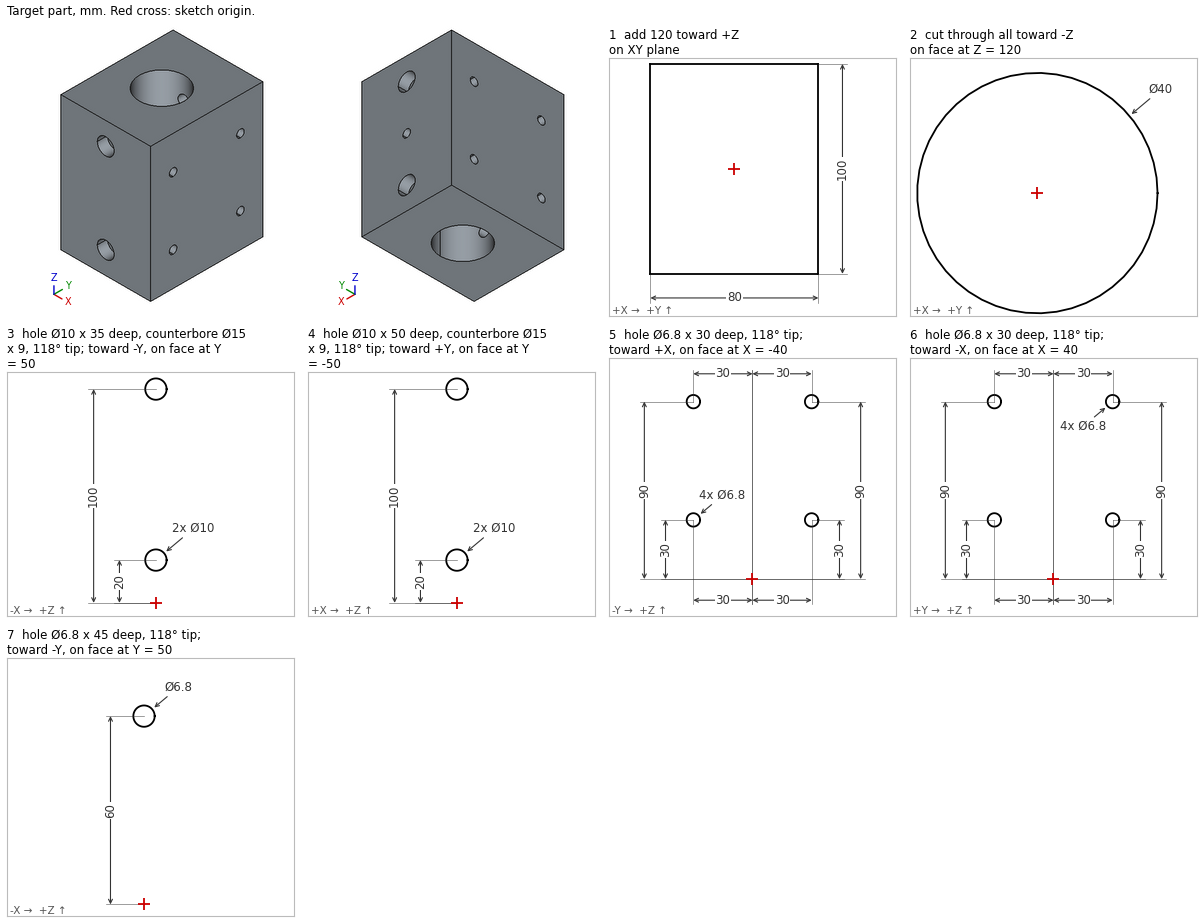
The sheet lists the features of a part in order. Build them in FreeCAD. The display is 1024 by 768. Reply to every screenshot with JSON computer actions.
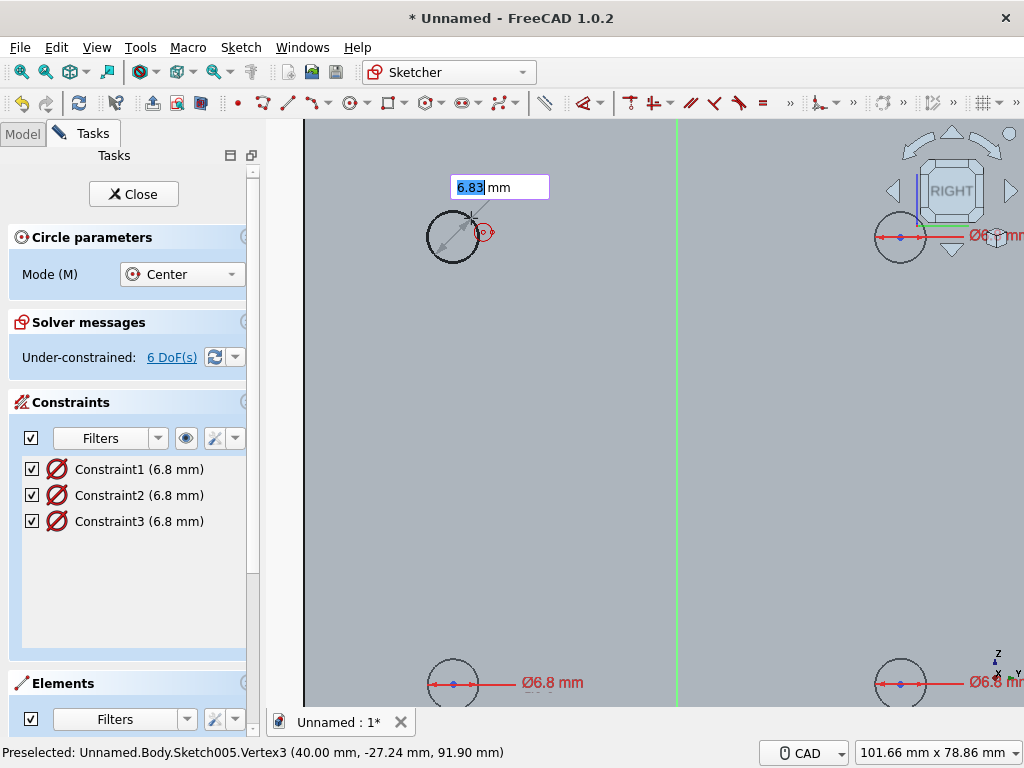
{"action": "type", "text": "6.8"}
{"action": "key", "text": "Return"}
{"action": "key", "text": "Escape"}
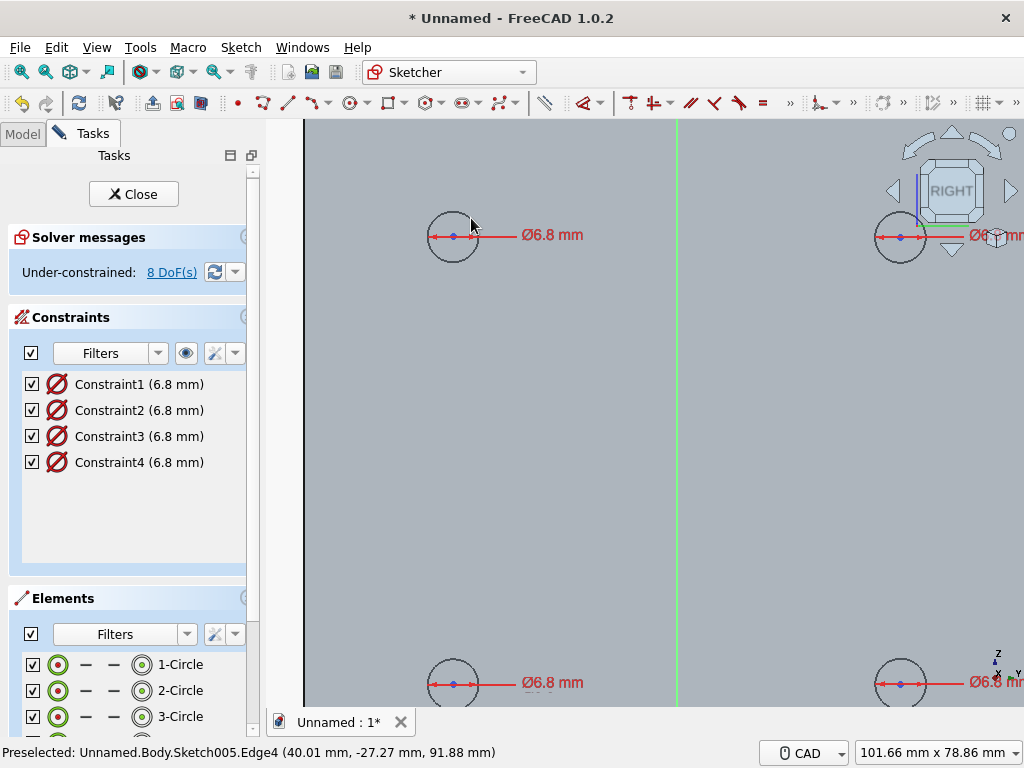
{"action": "left_click", "coordinate": [584, 104]}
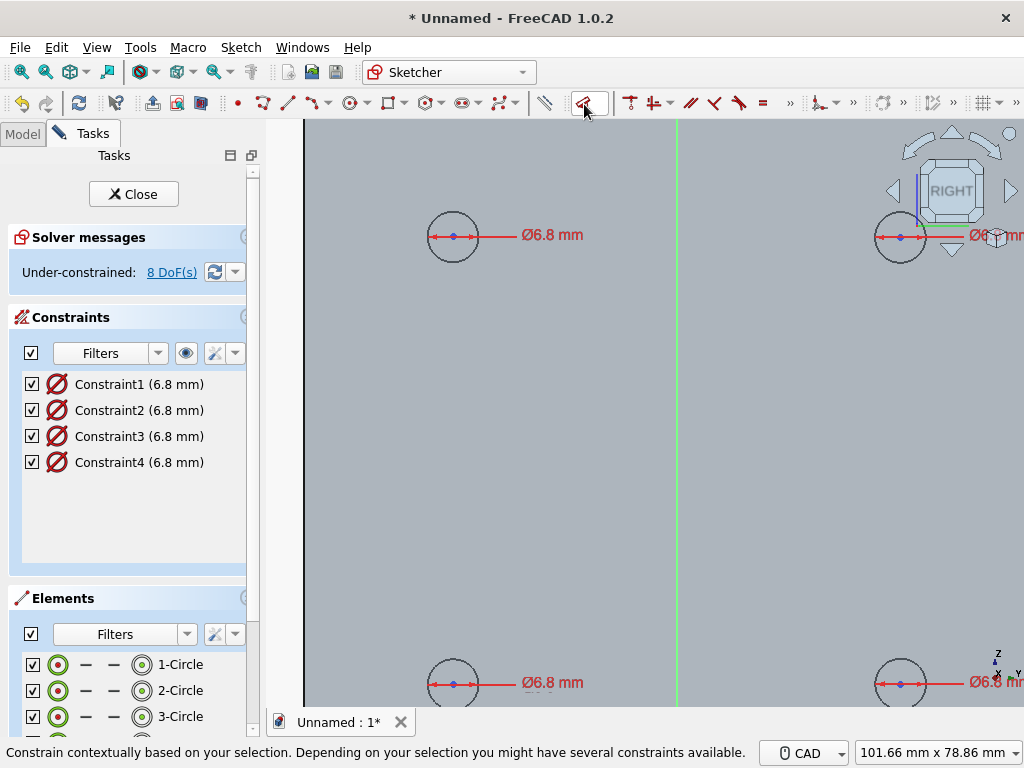
{"action": "scroll", "coordinate": [454, 235], "scroll_direction": "down", "scroll_amount": 3}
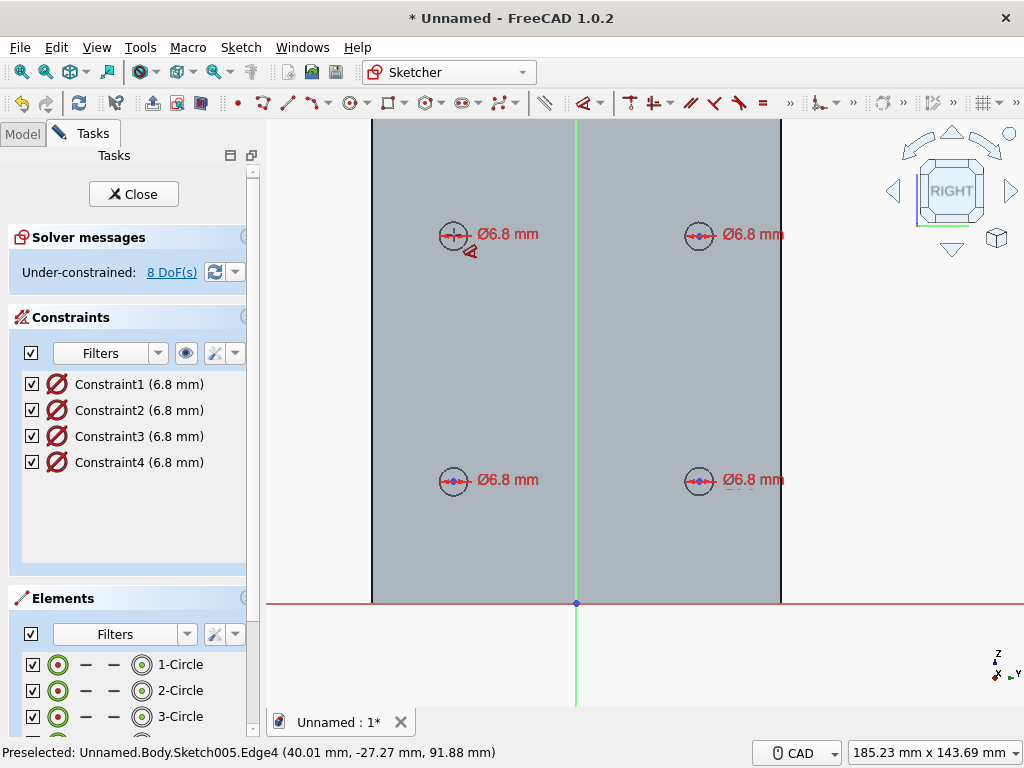
{"action": "left_click", "coordinate": [699, 236]}
{"action": "left_click", "coordinate": [638, 638]}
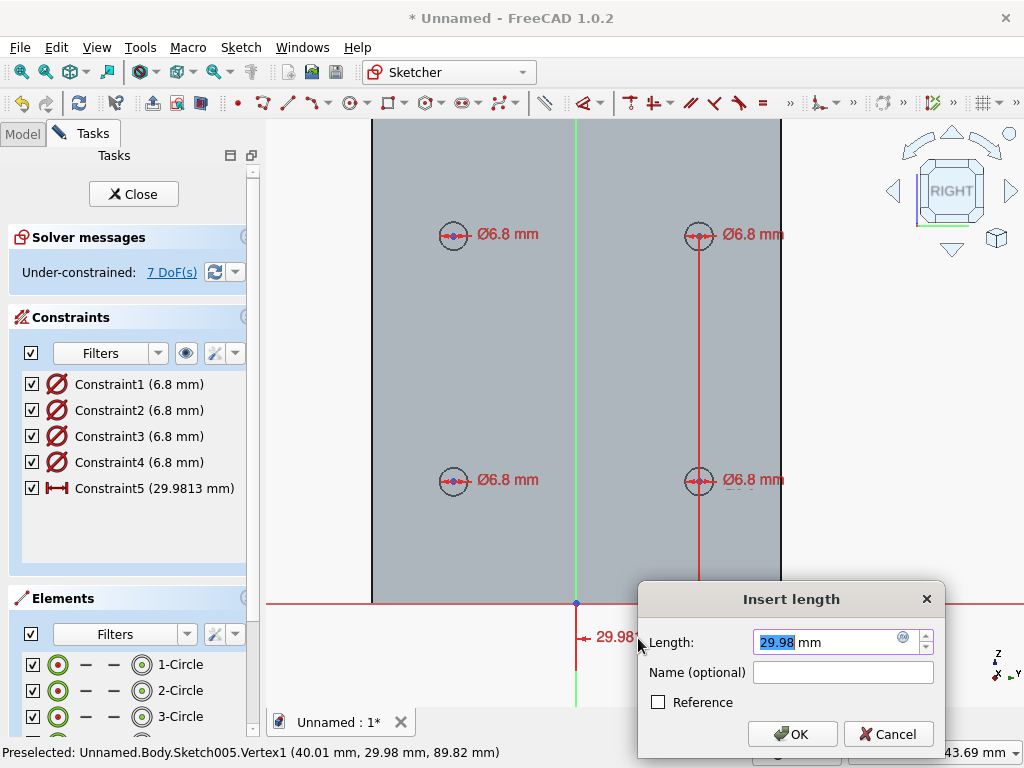
{"action": "type", "text": "30"}
{"action": "key", "text": "Return"}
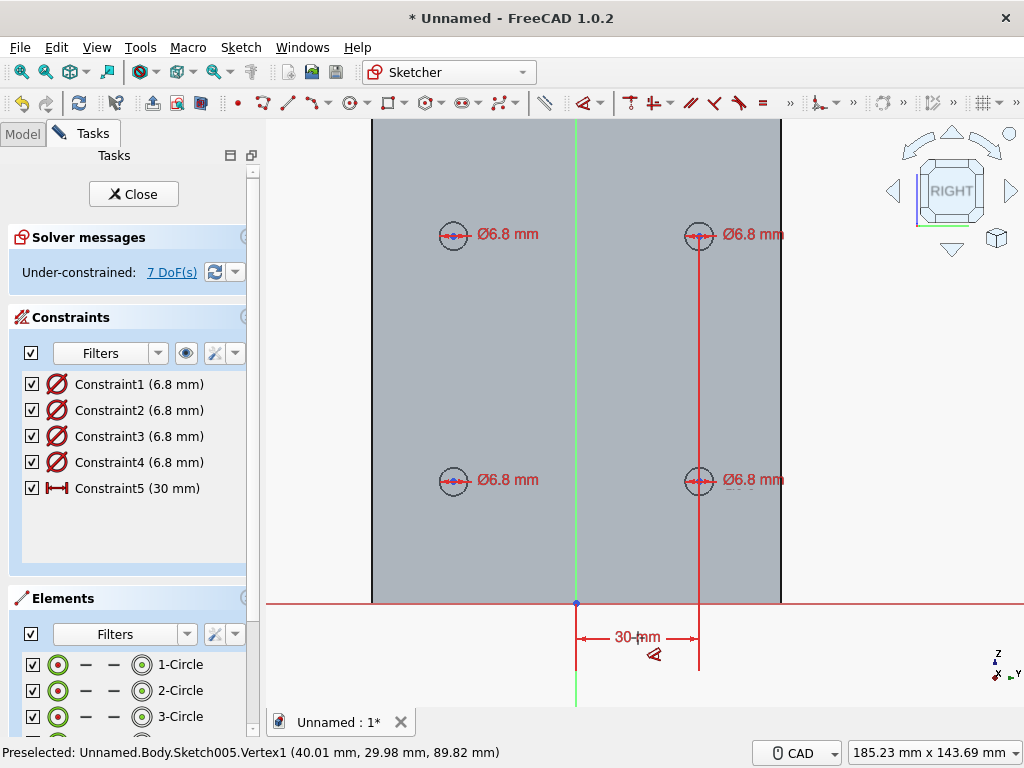
{"action": "left_click", "coordinate": [699, 236]}
{"action": "left_click", "coordinate": [733, 420]}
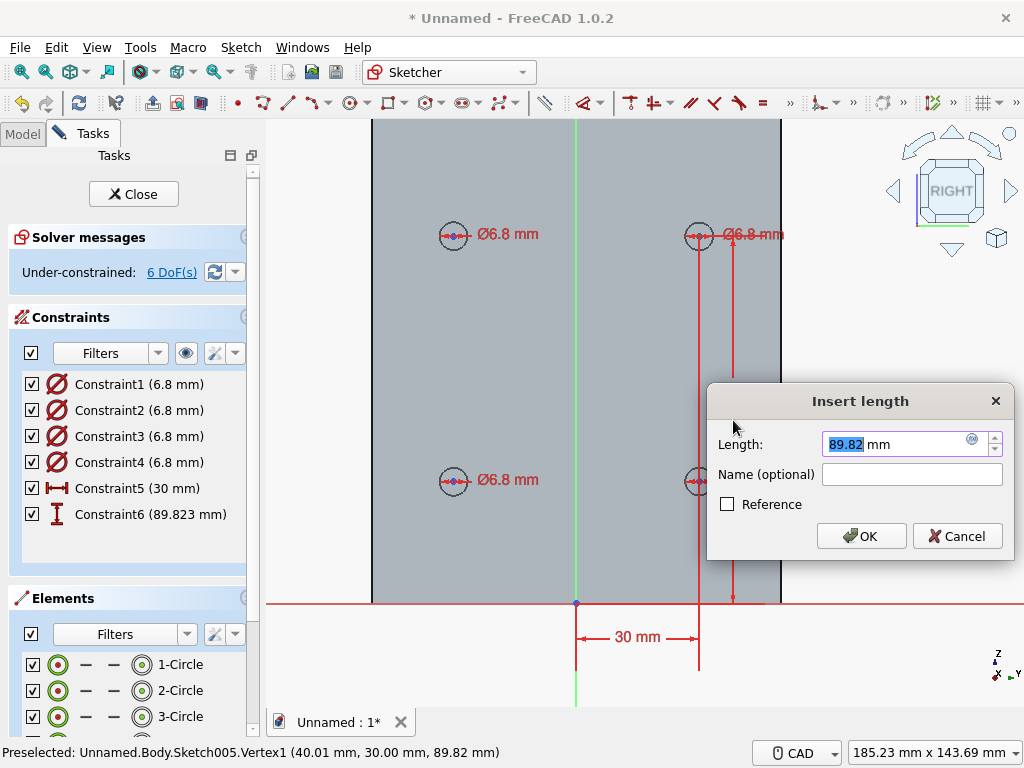
{"action": "type", "text": "90"}
{"action": "key", "text": "Return"}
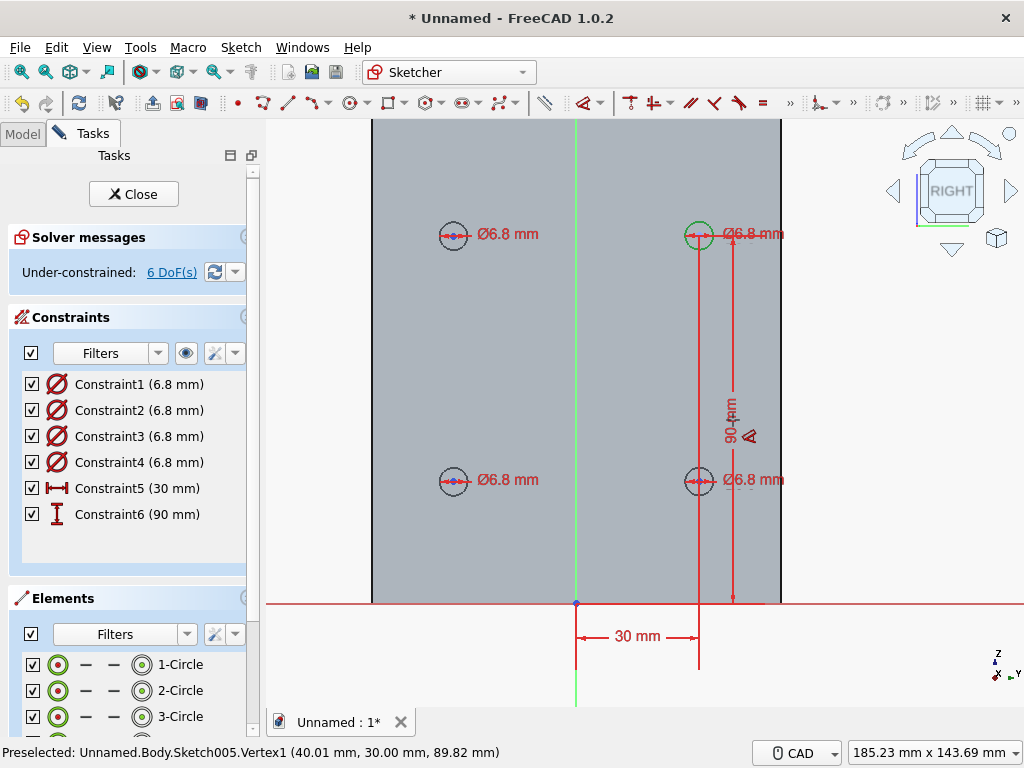
{"action": "left_click", "coordinate": [699, 482]}
{"action": "left_click", "coordinate": [638, 448]}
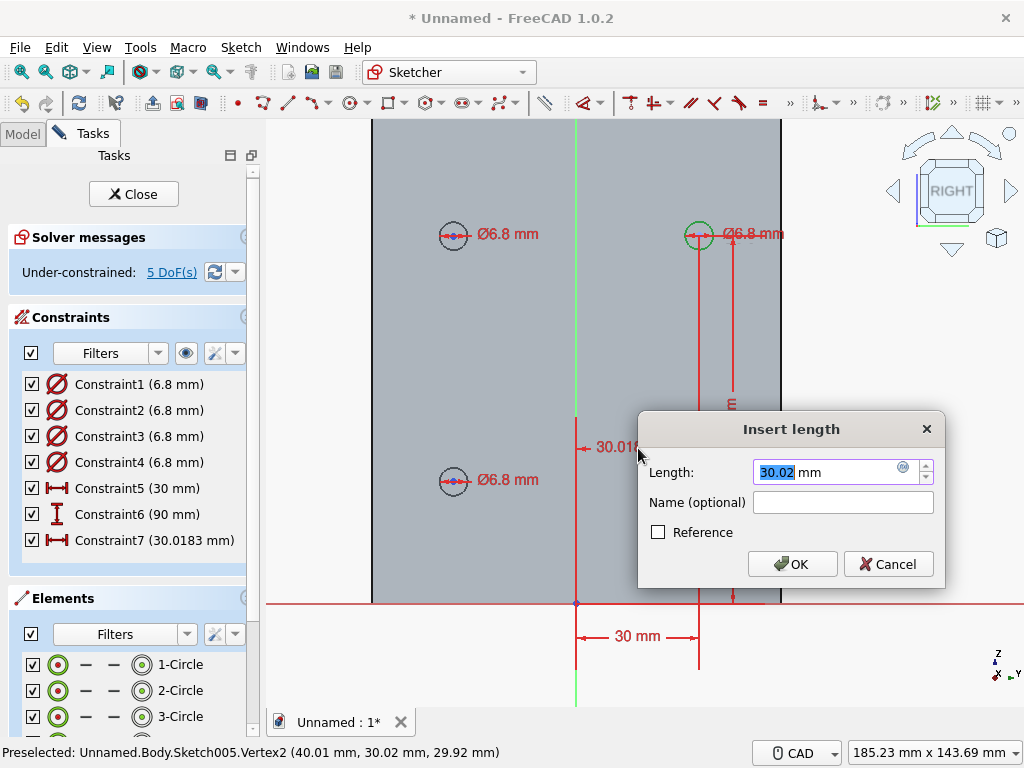
{"action": "type", "text": "30"}
{"action": "key", "text": "Return"}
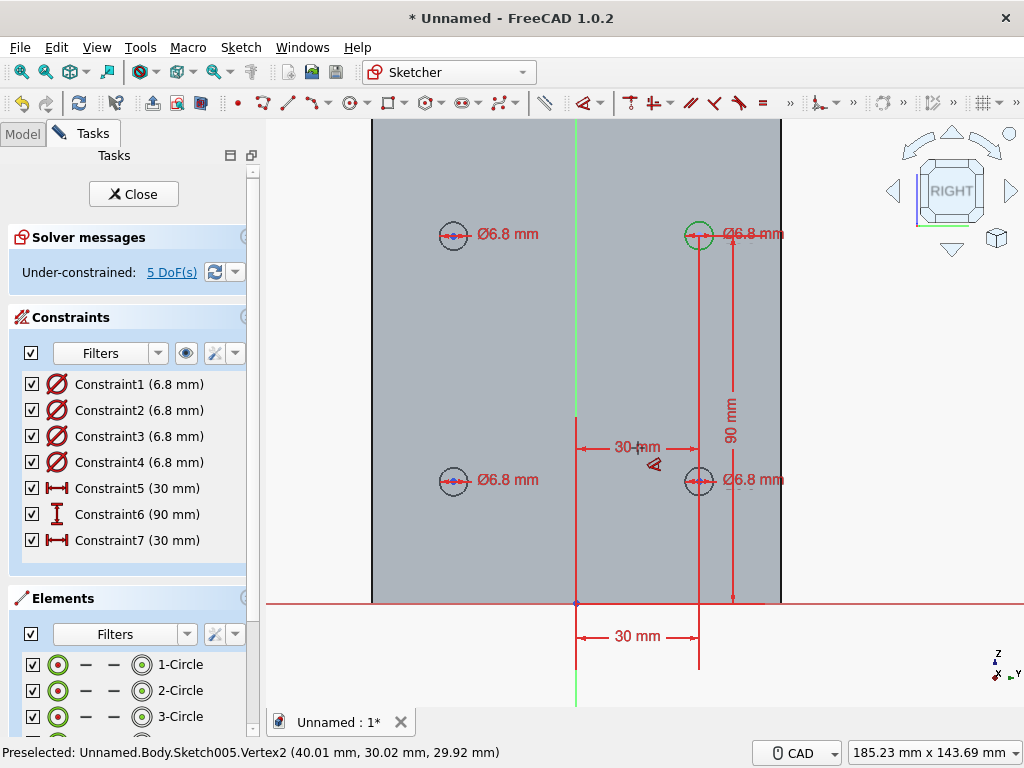
{"action": "left_click", "coordinate": [699, 482]}
{"action": "left_click", "coordinate": [733, 543]}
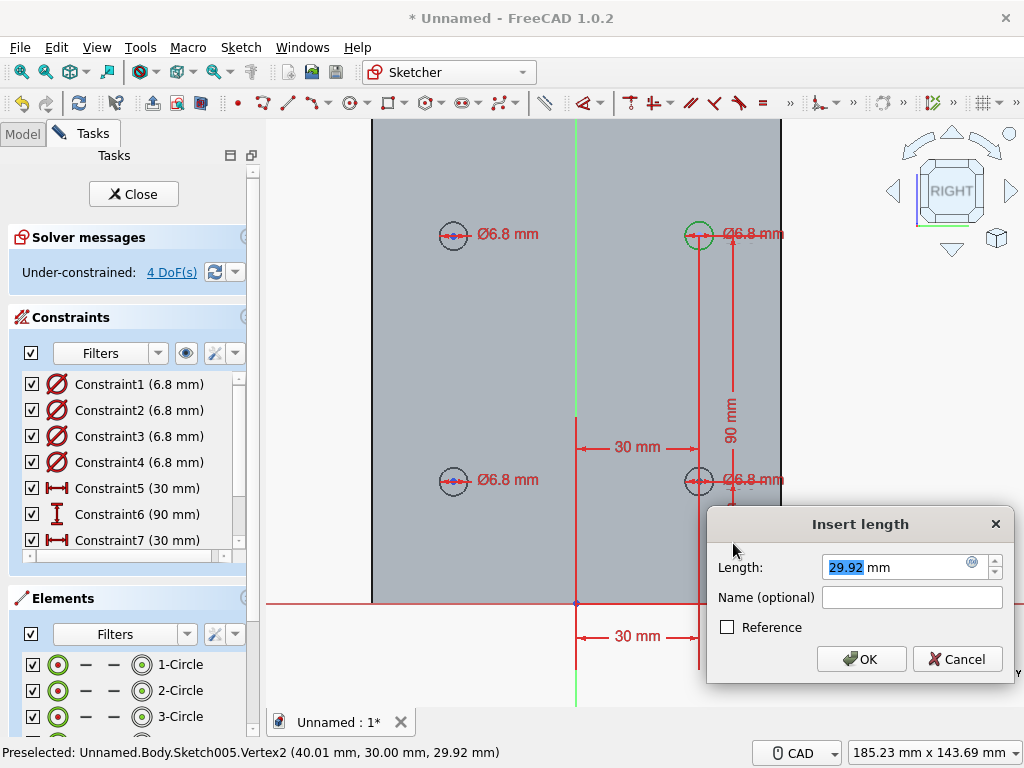
{"action": "type", "text": "30"}
{"action": "key", "text": "Return"}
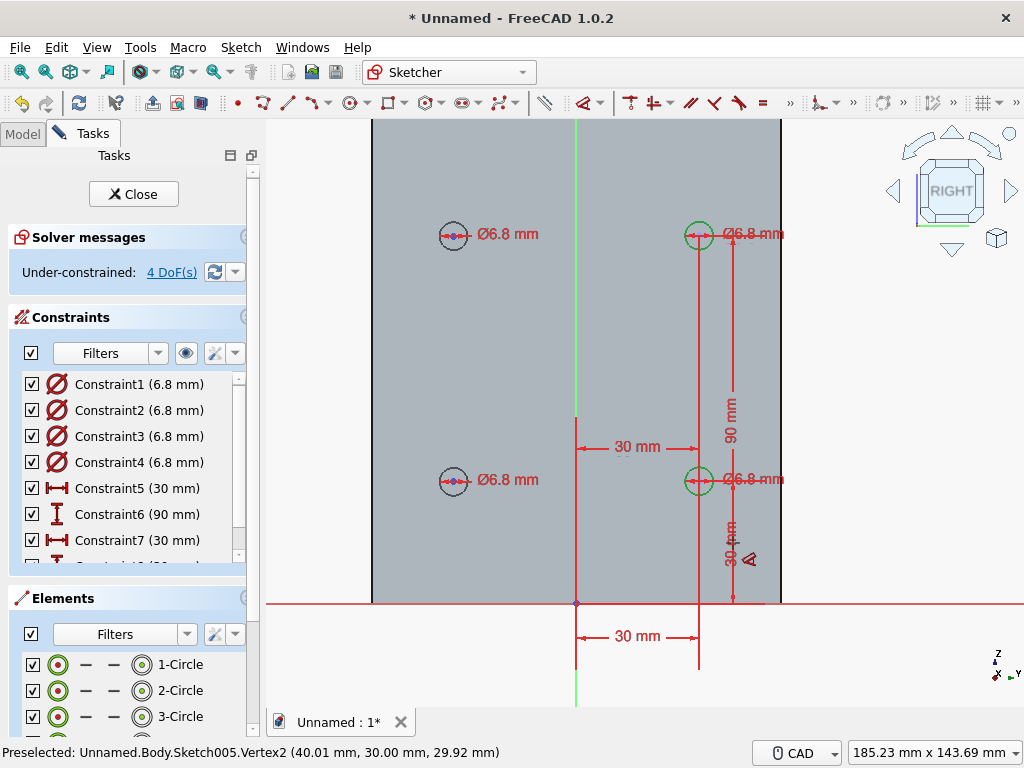
{"action": "left_click", "coordinate": [454, 482]}
{"action": "left_click", "coordinate": [515, 638]}